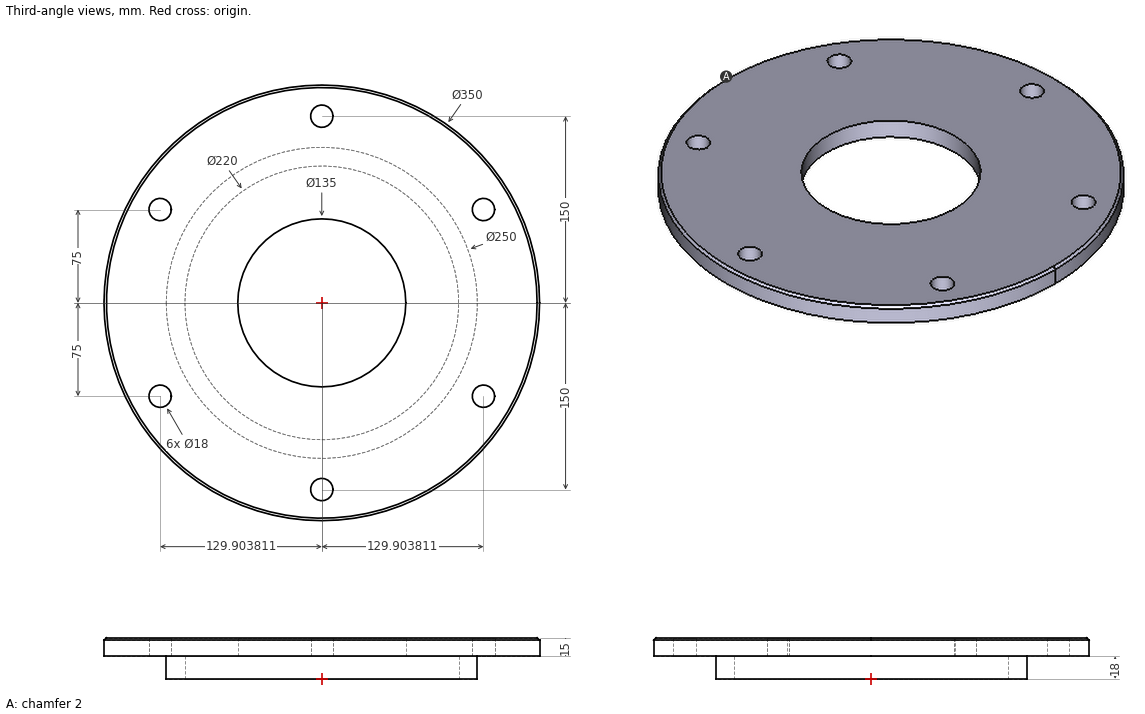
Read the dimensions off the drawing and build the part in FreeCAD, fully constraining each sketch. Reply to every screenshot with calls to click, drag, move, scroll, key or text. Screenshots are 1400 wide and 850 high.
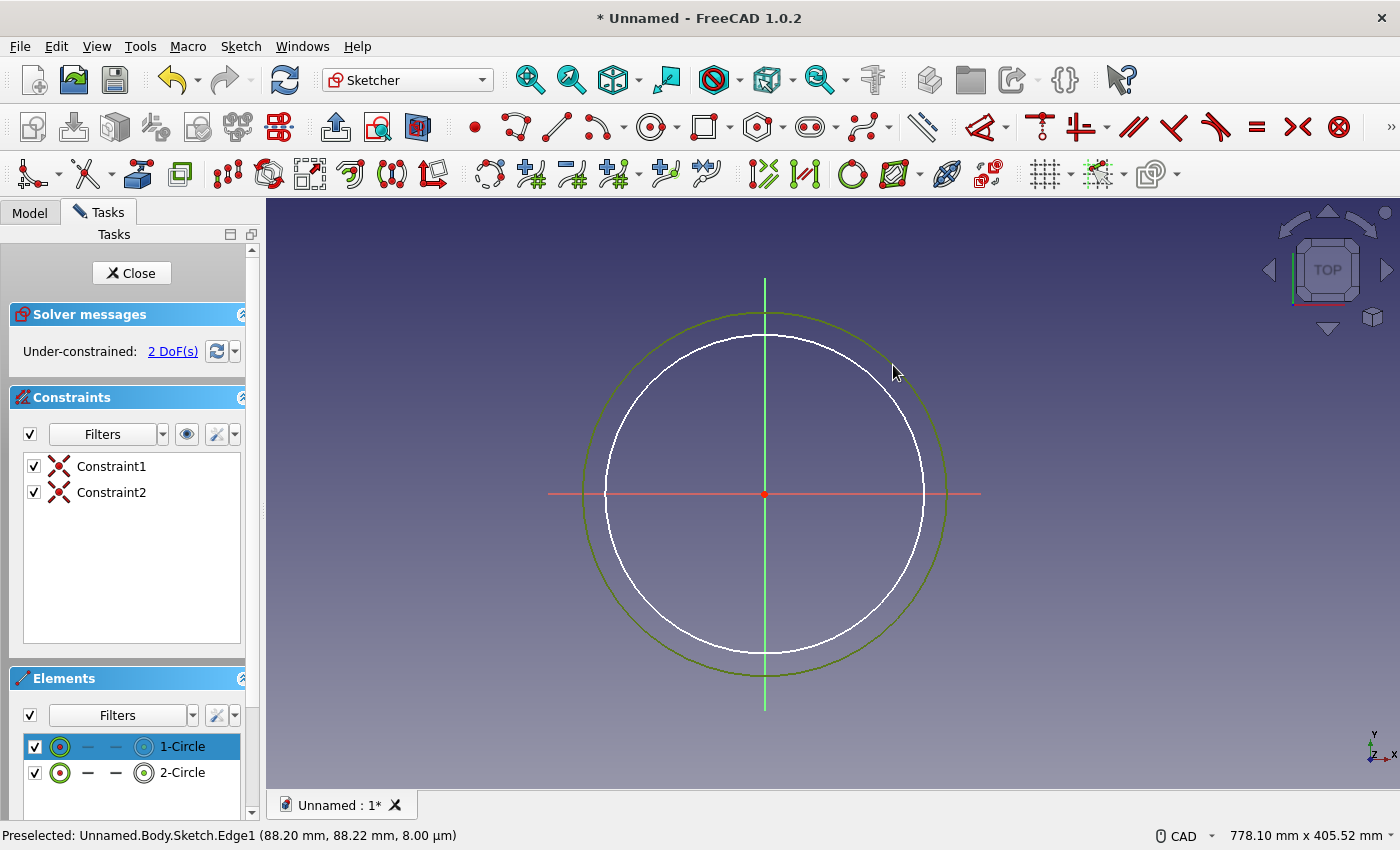
click(1006, 128)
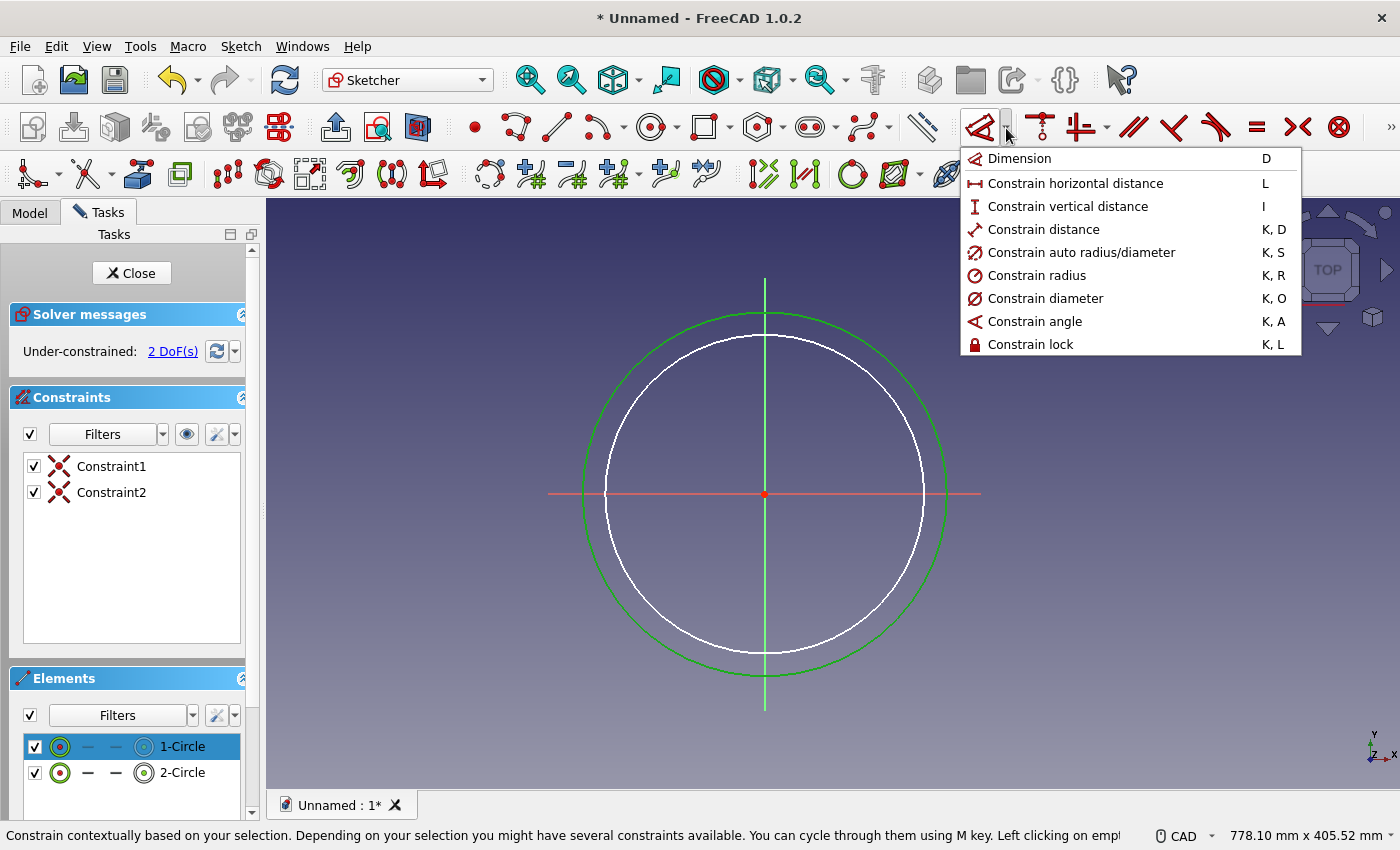
click(1131, 298)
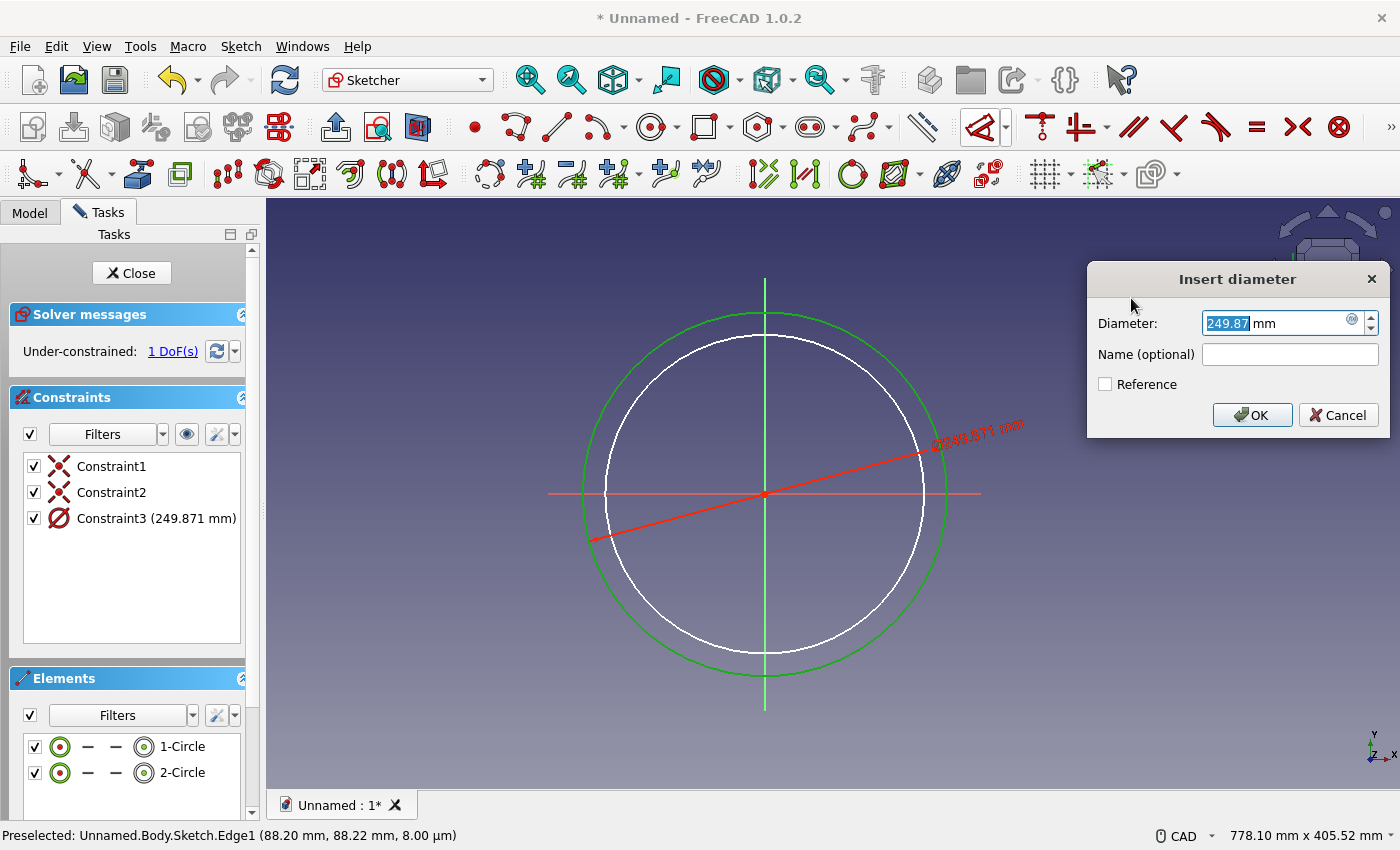
text(250)
key(Return)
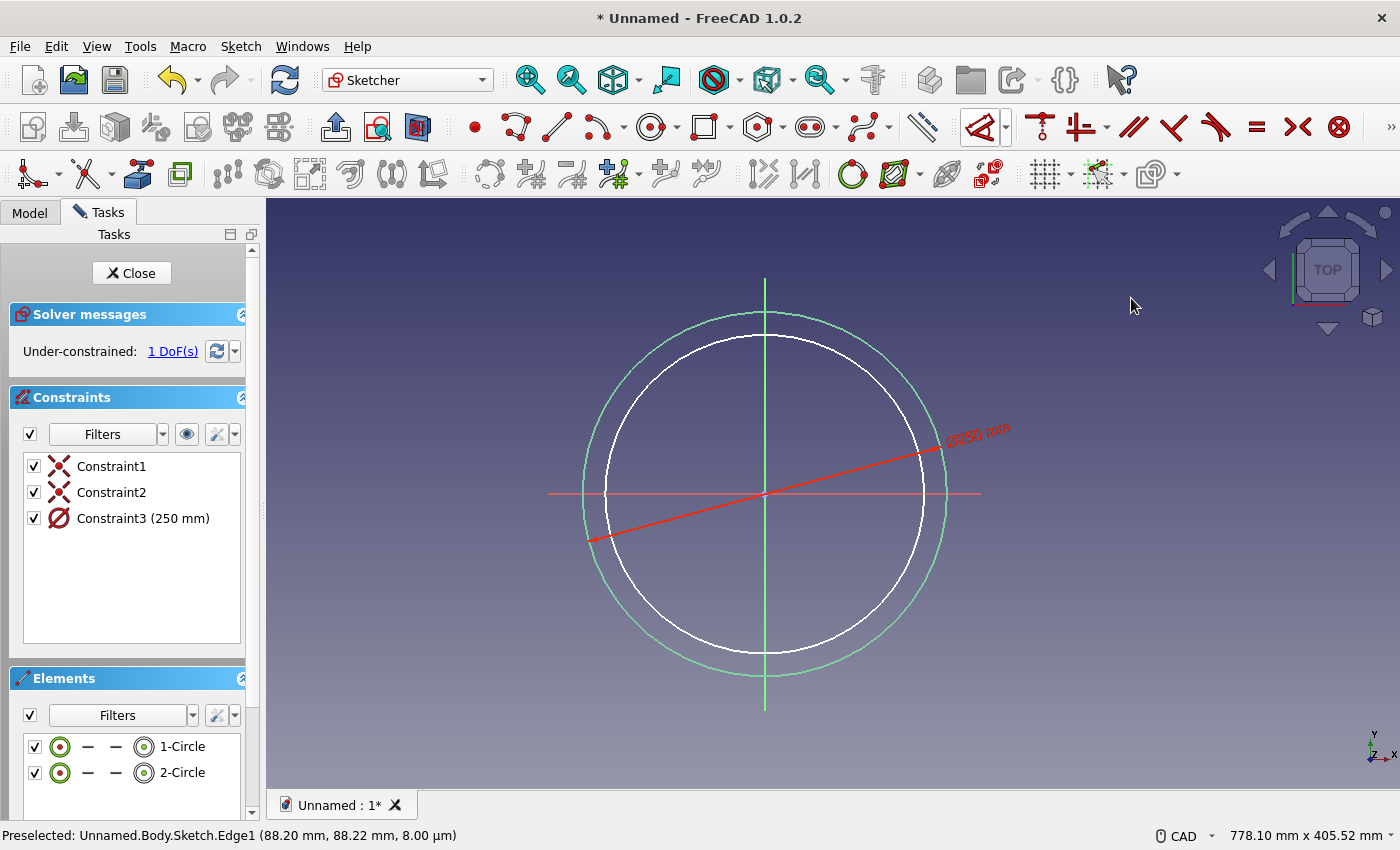
click(877, 381)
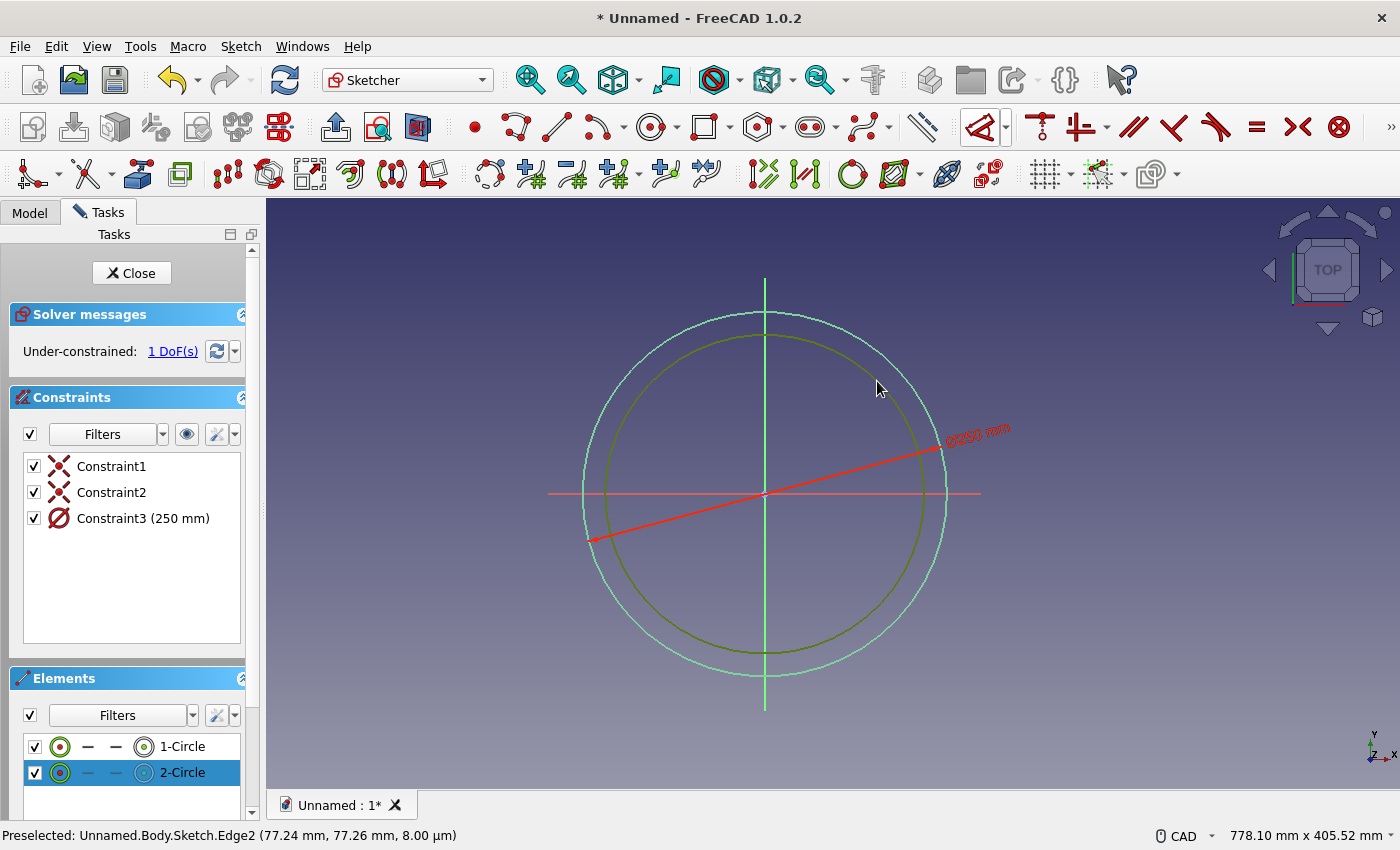
click(1006, 128)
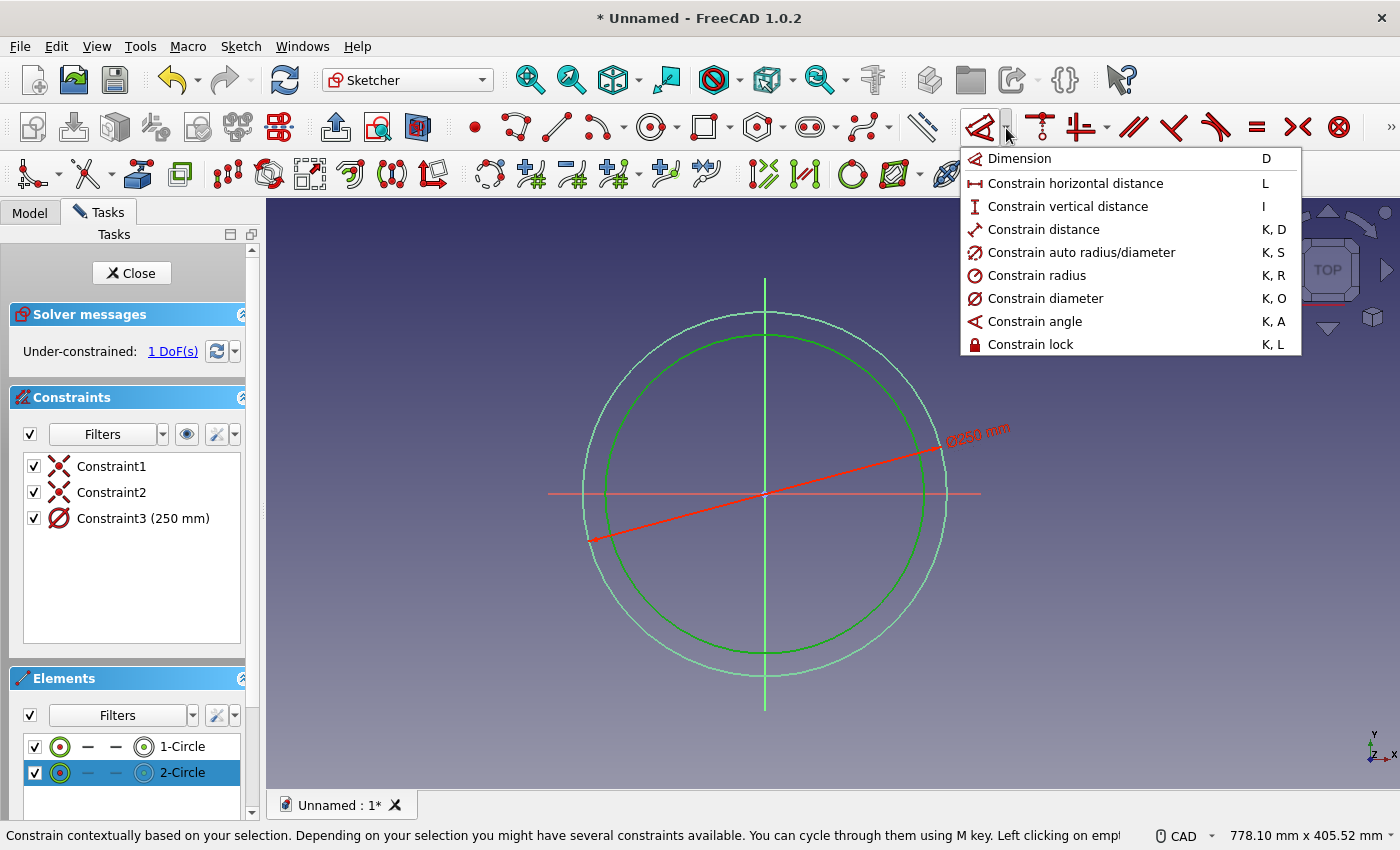
click(1131, 298)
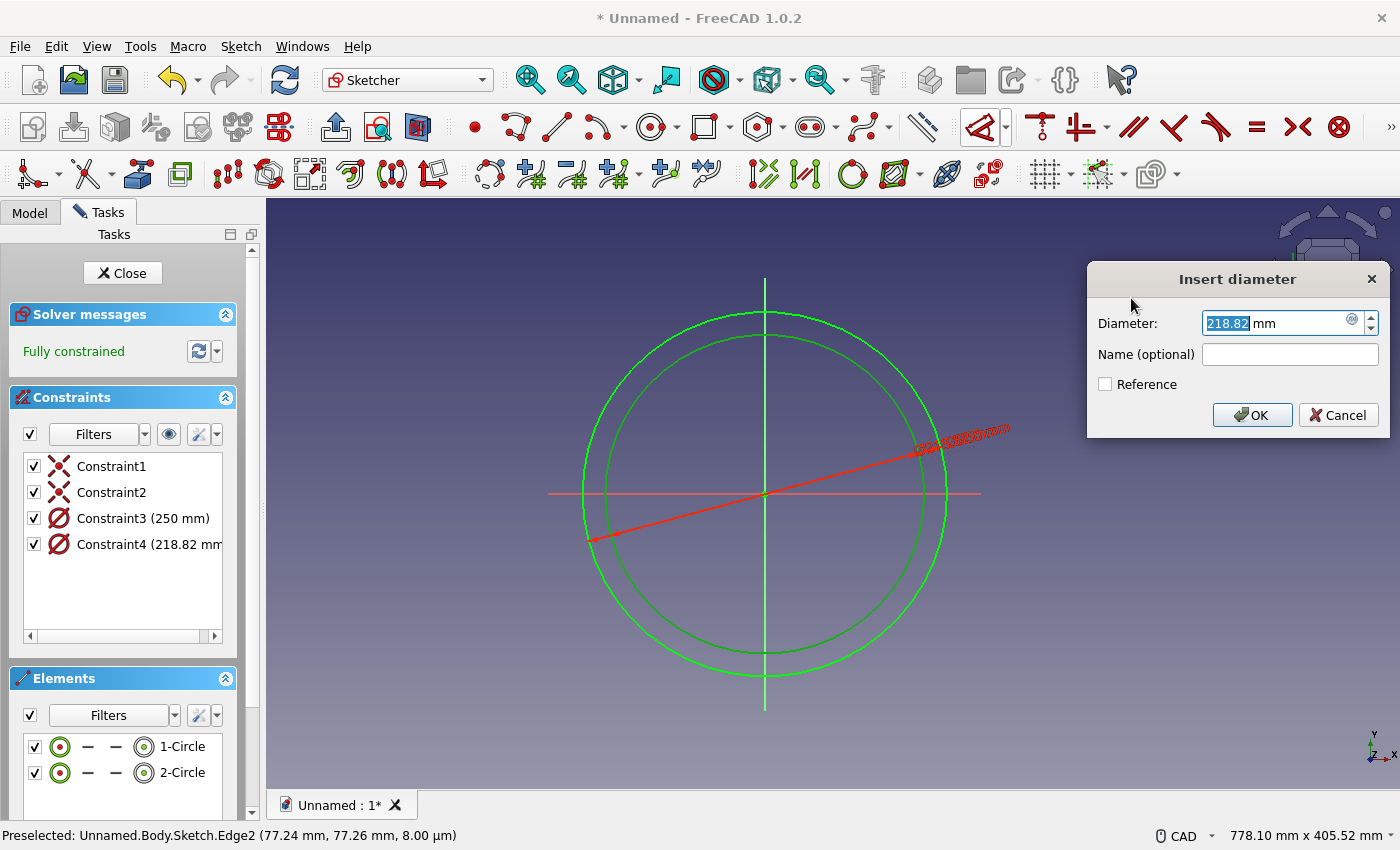
text(220)
key(Return)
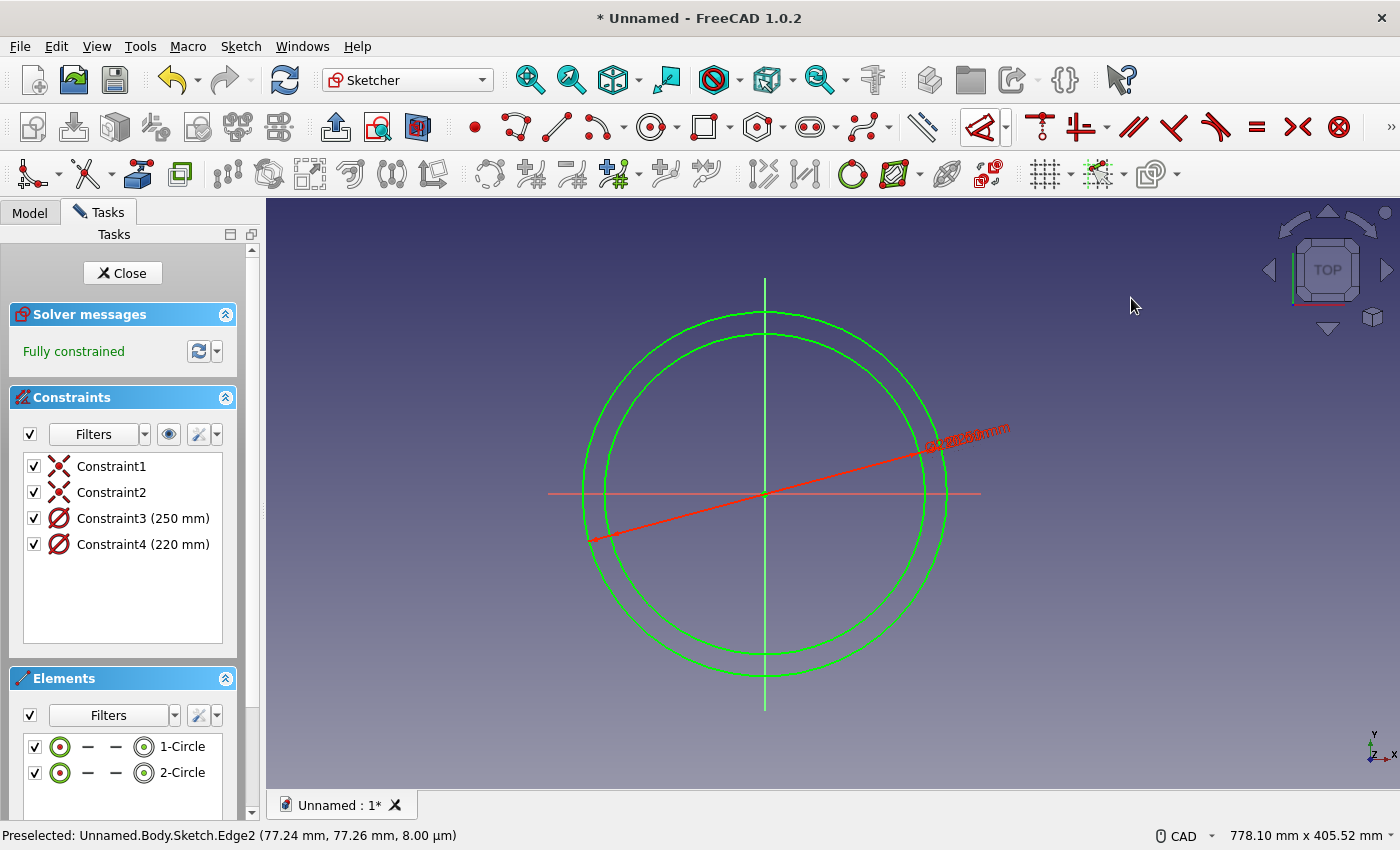
click(123, 273)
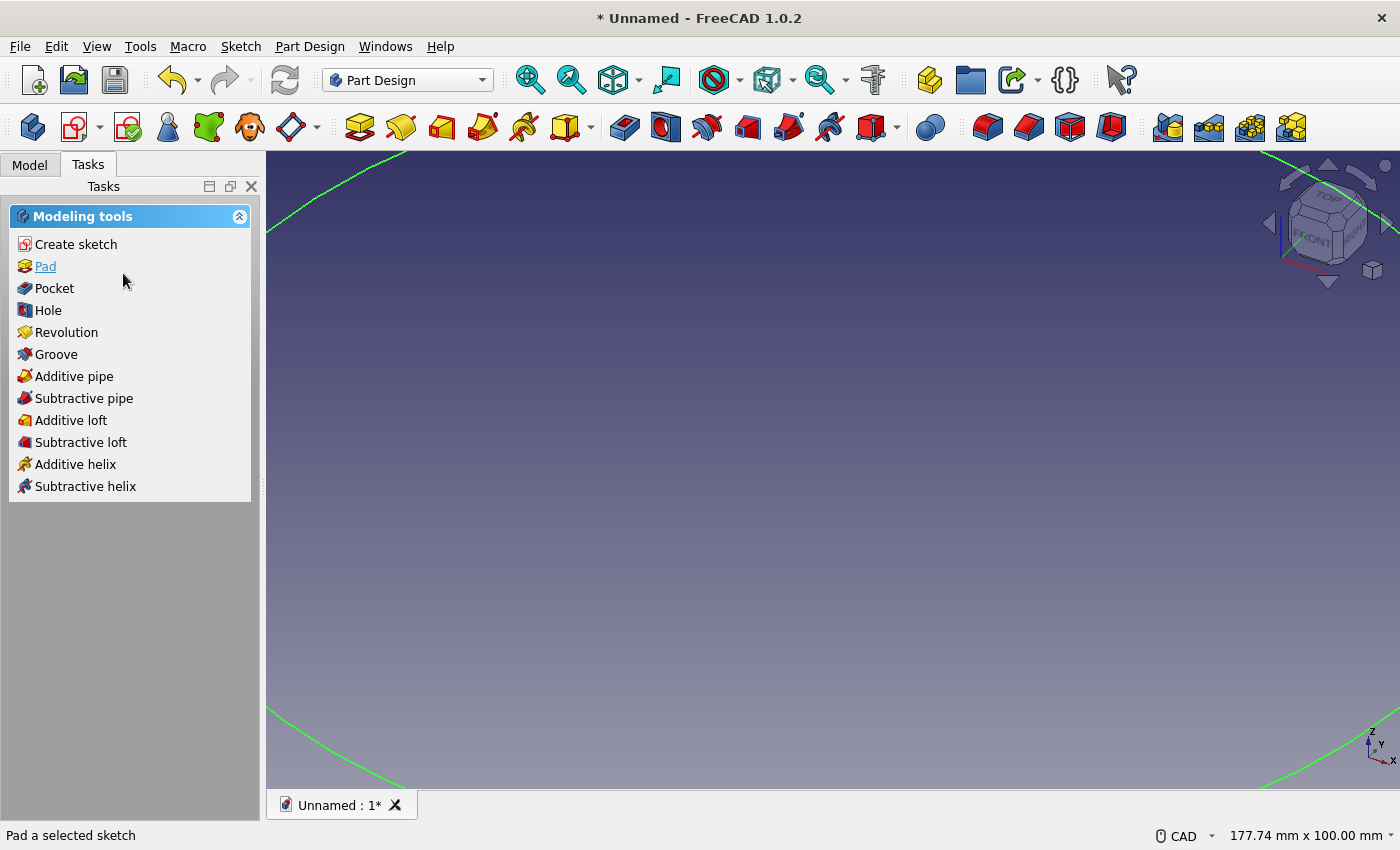
click(360, 128)